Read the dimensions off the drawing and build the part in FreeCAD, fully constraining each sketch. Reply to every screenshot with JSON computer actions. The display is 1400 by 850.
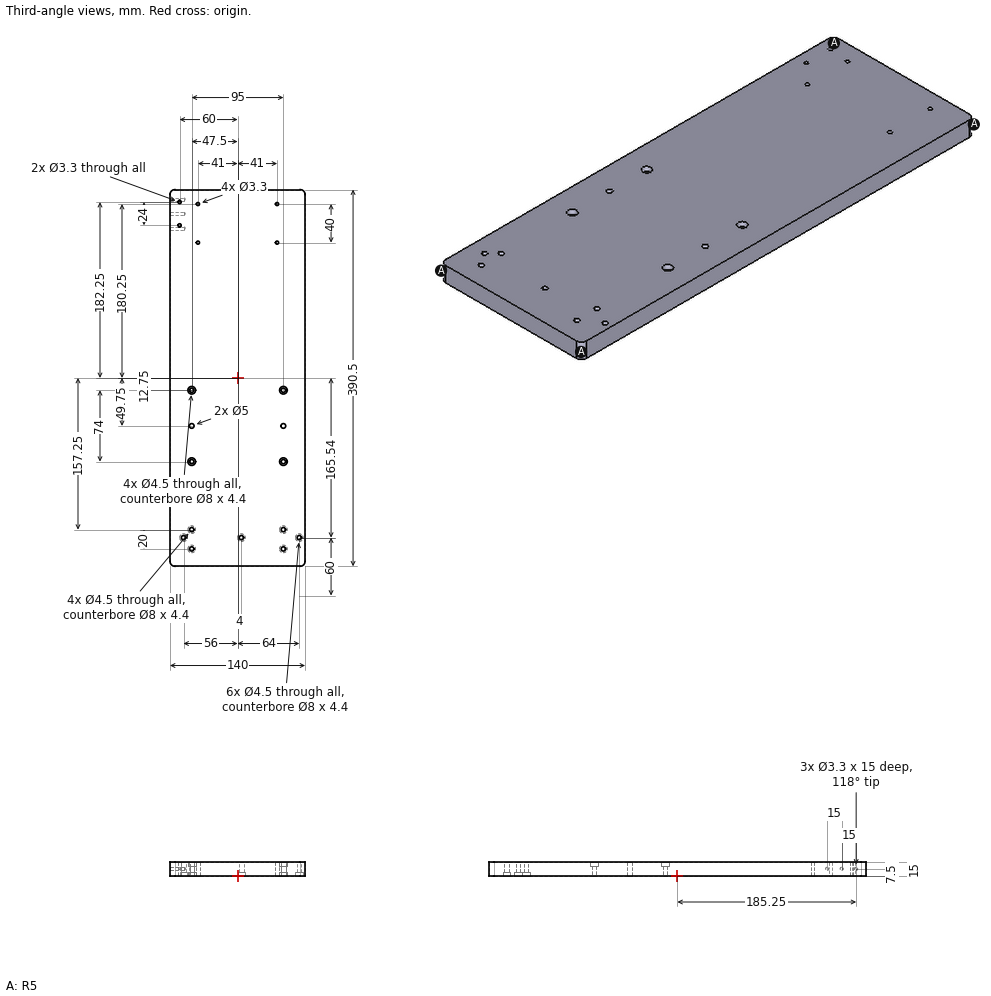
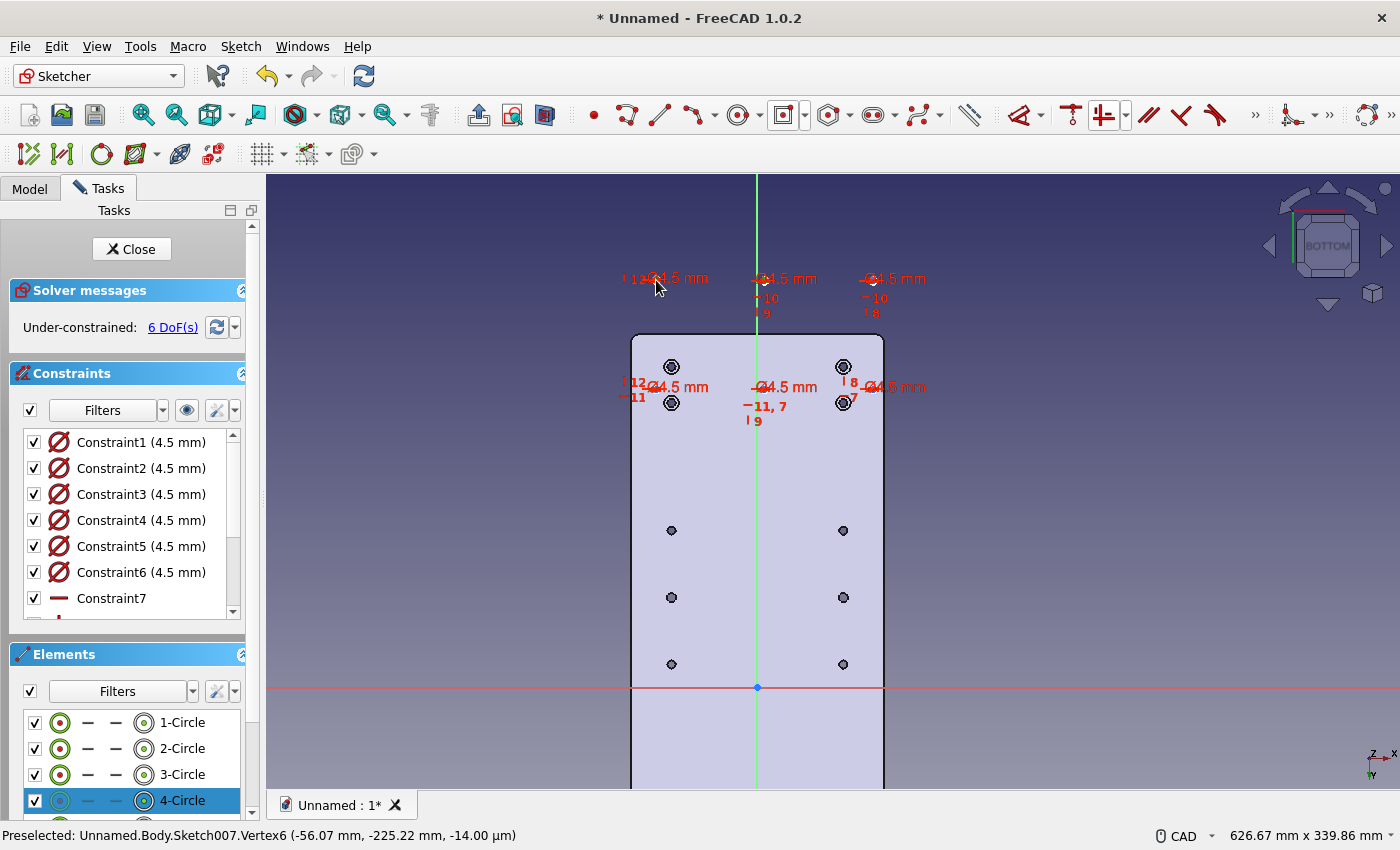
{"action": "left_click", "coordinate": [1126, 116]}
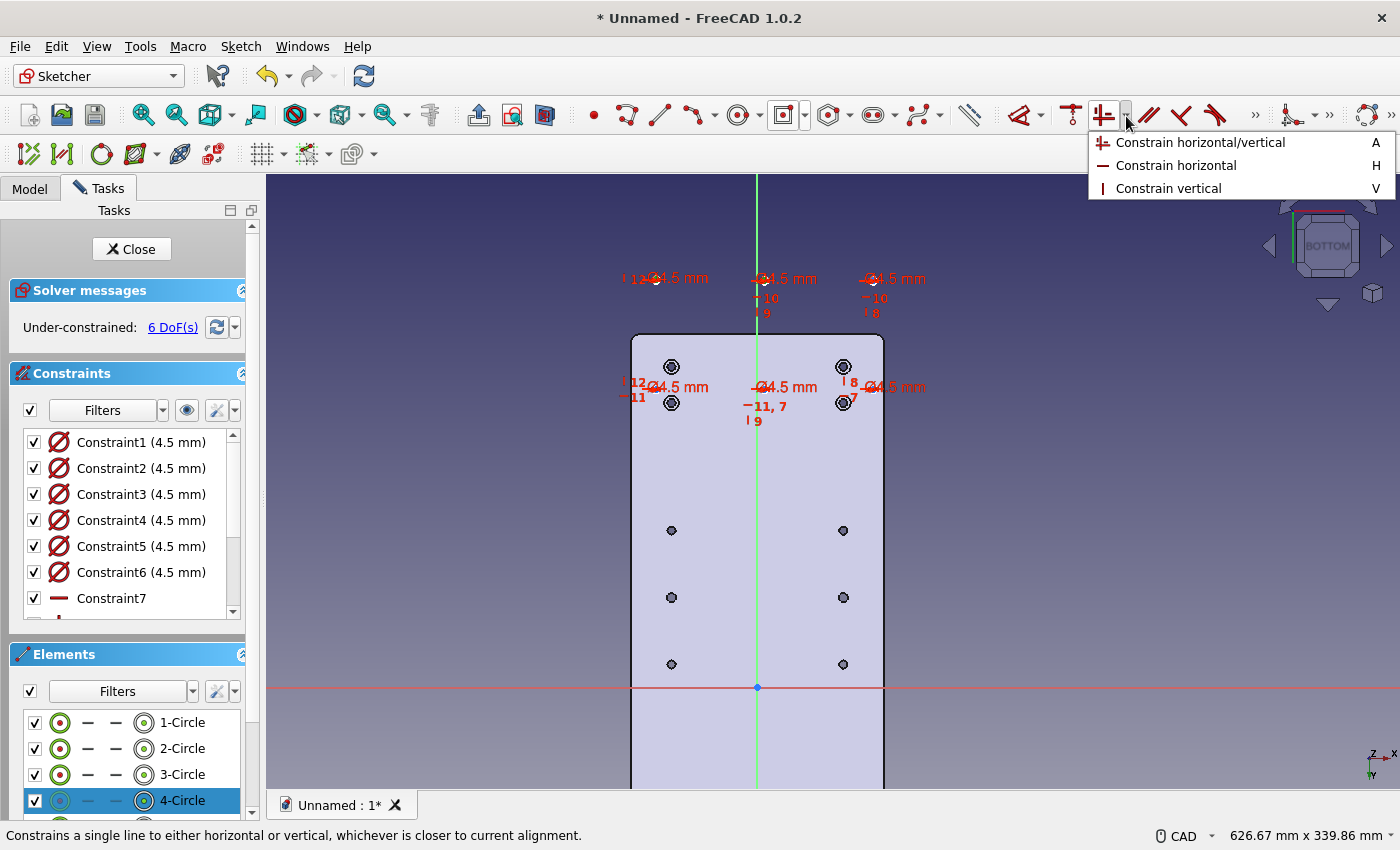
{"action": "left_click", "coordinate": [1242, 166]}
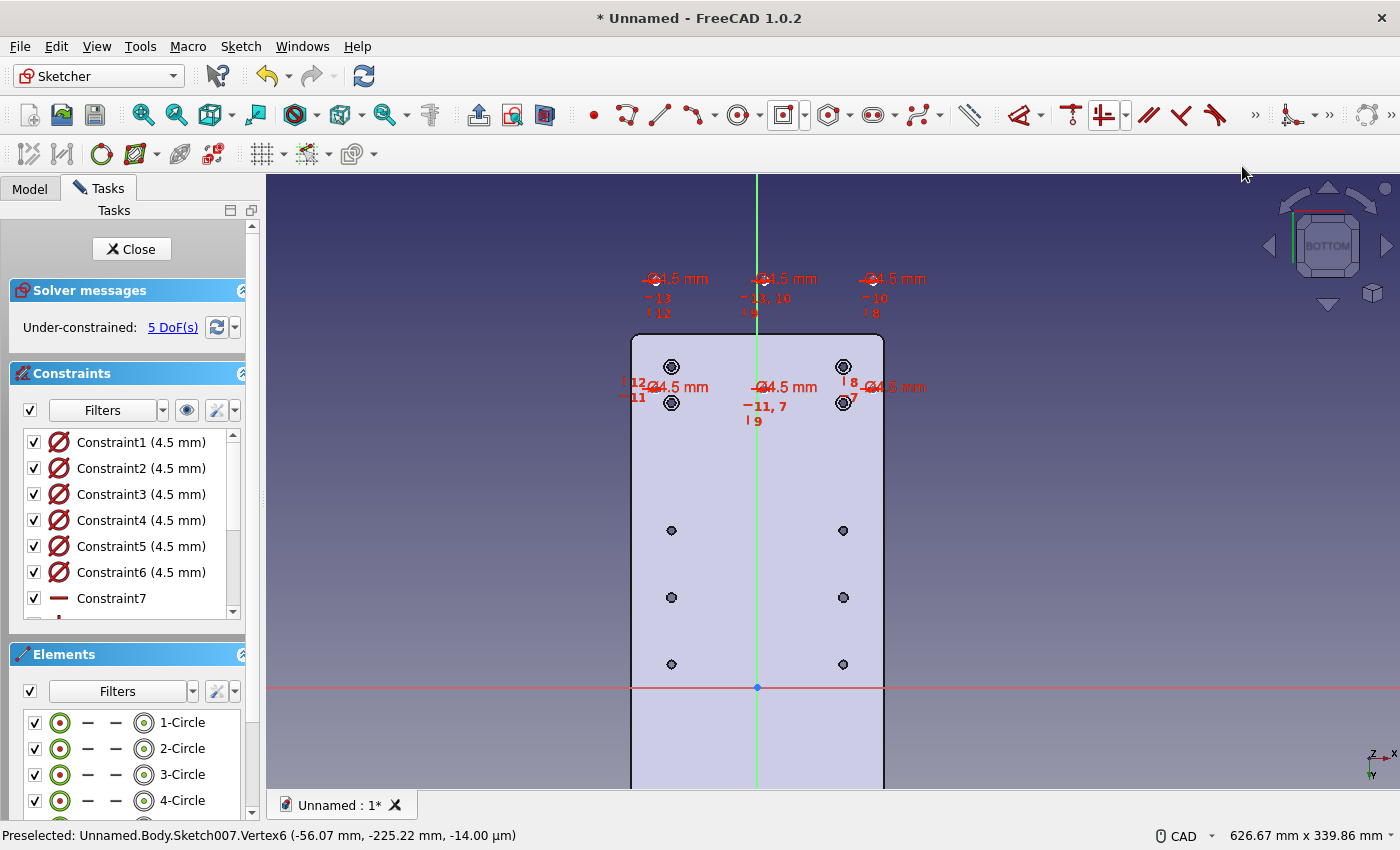
{"action": "left_click", "coordinate": [1018, 116]}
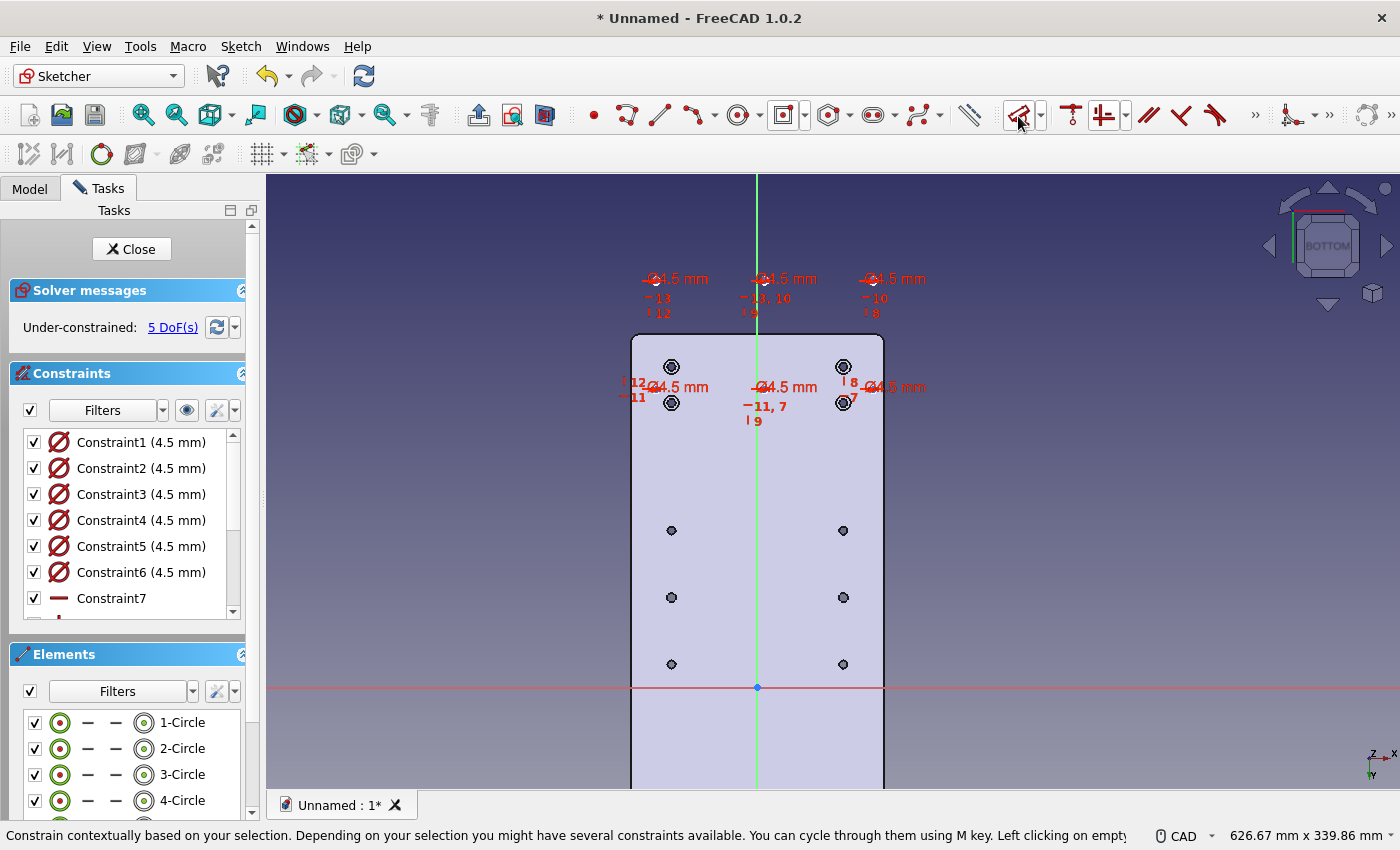
{"action": "scroll", "coordinate": [765, 389], "scroll_direction": "up", "scroll_amount": 9}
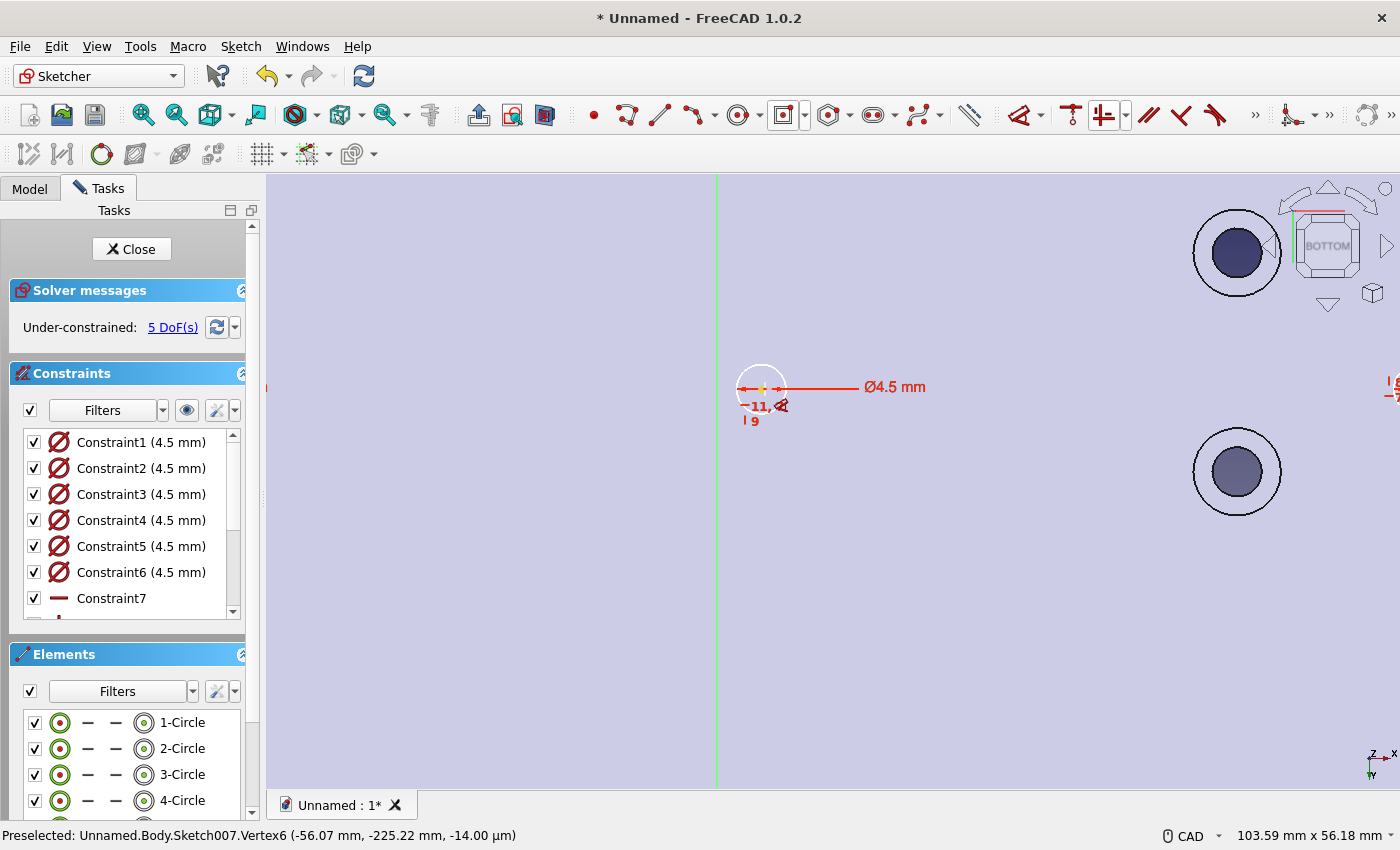
{"action": "left_click", "coordinate": [761, 389]}
{"action": "left_click", "coordinate": [739, 355]}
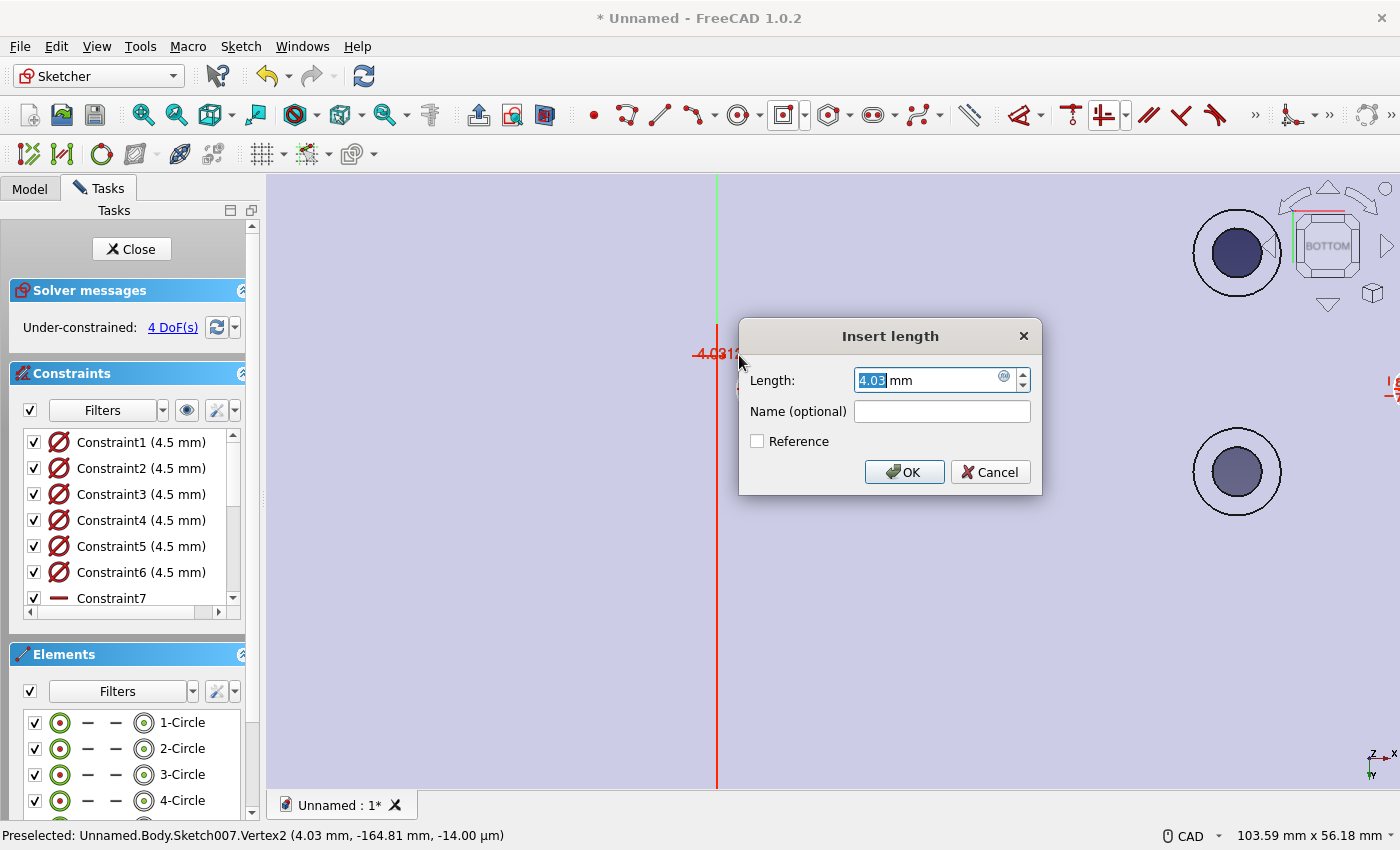
{"action": "type", "text": "4"}
{"action": "key", "text": "Return"}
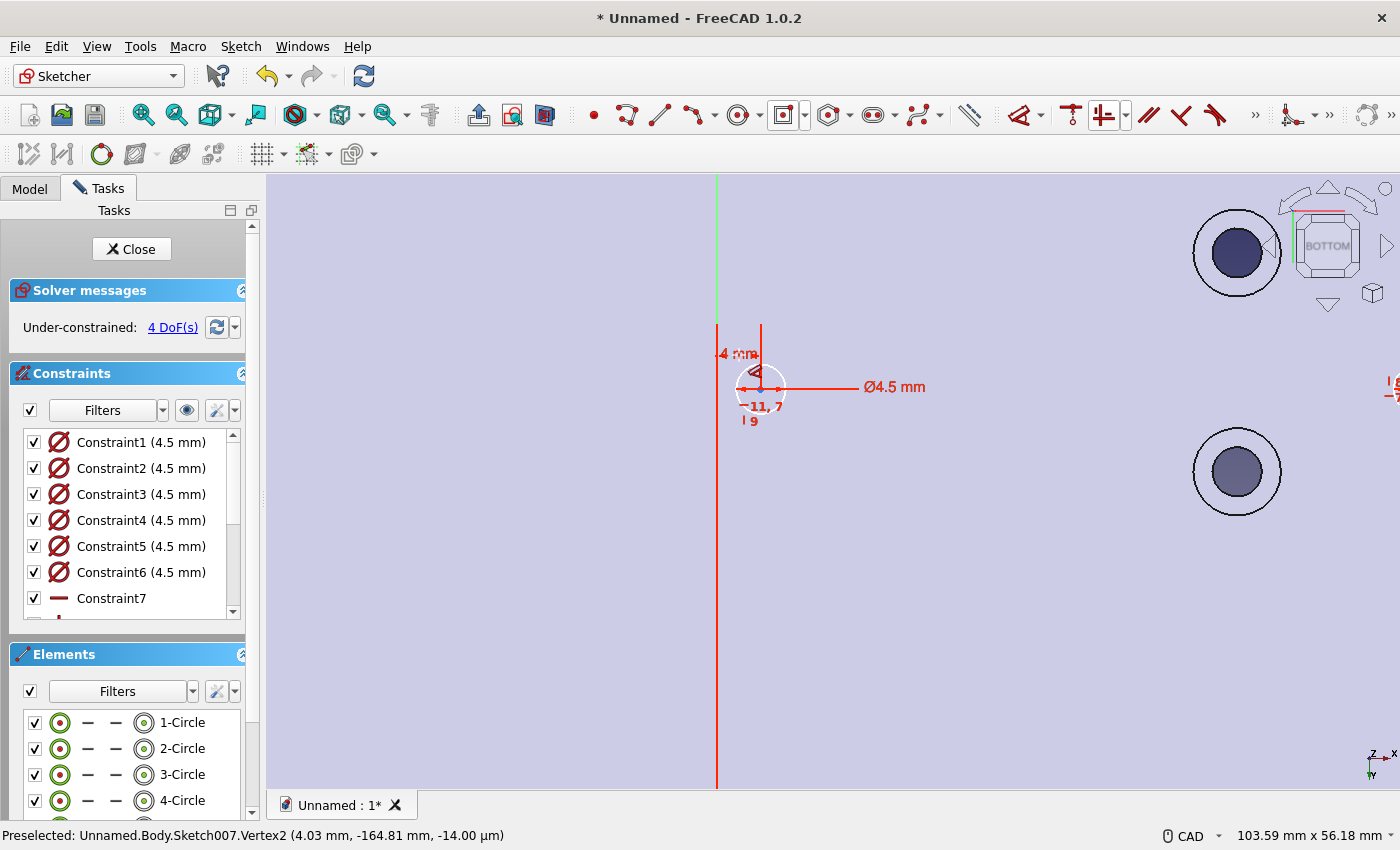
{"action": "scroll", "coordinate": [765, 389], "scroll_direction": "down", "scroll_amount": 9}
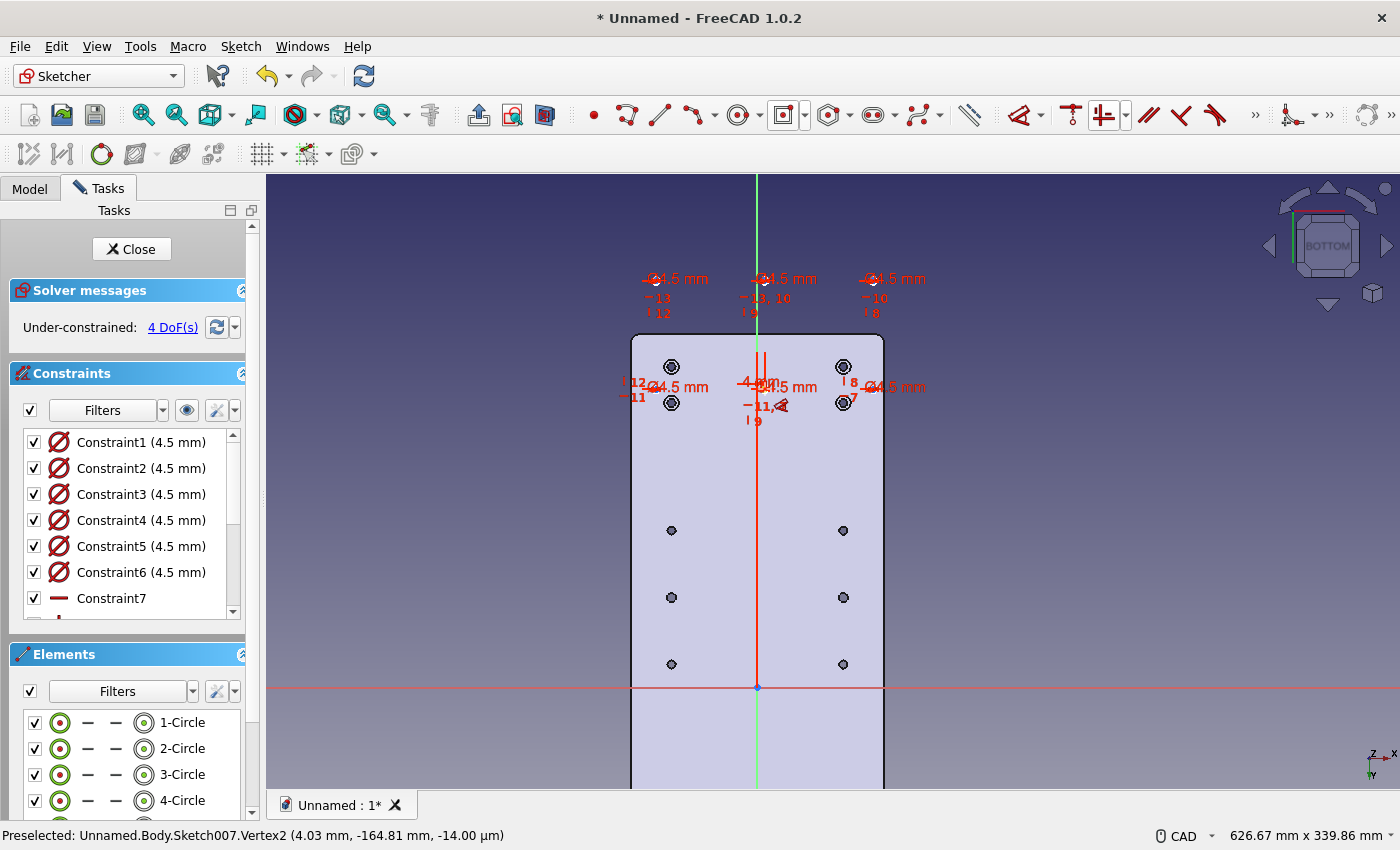
{"action": "left_click", "coordinate": [873, 389]}
{"action": "left_click", "coordinate": [815, 722]}